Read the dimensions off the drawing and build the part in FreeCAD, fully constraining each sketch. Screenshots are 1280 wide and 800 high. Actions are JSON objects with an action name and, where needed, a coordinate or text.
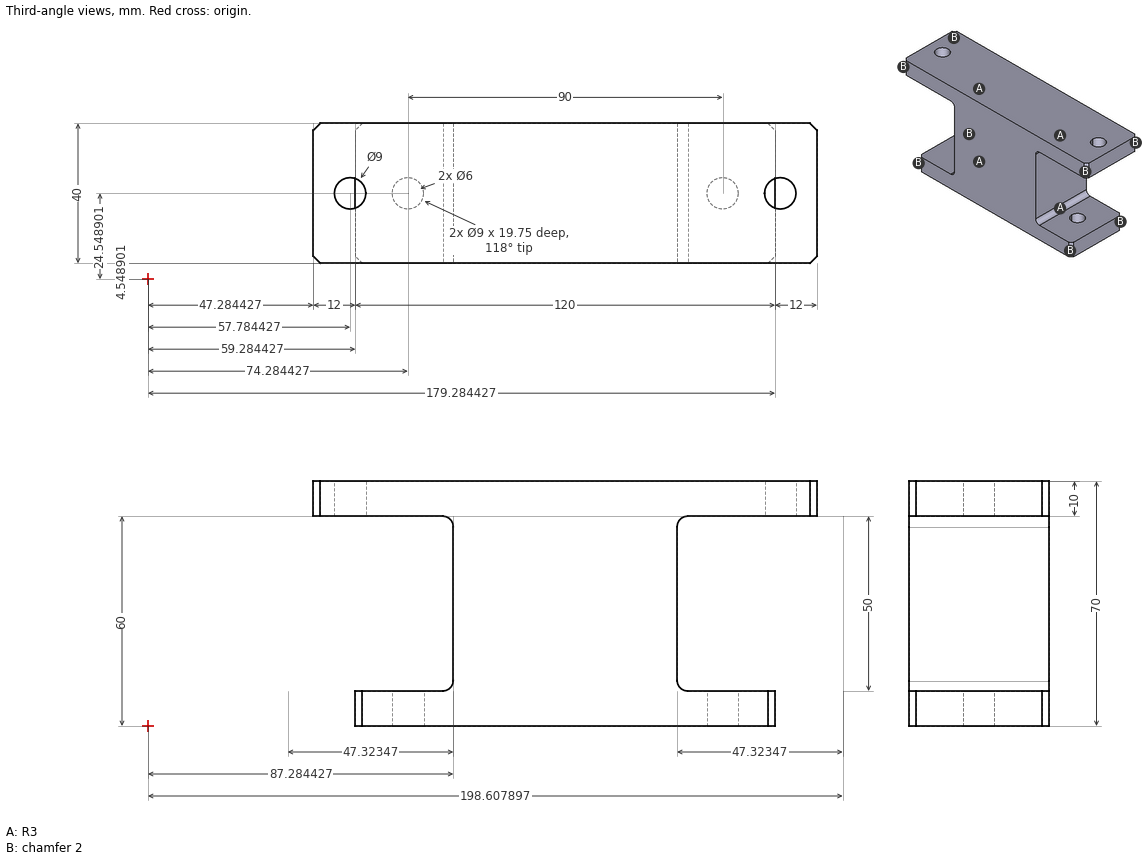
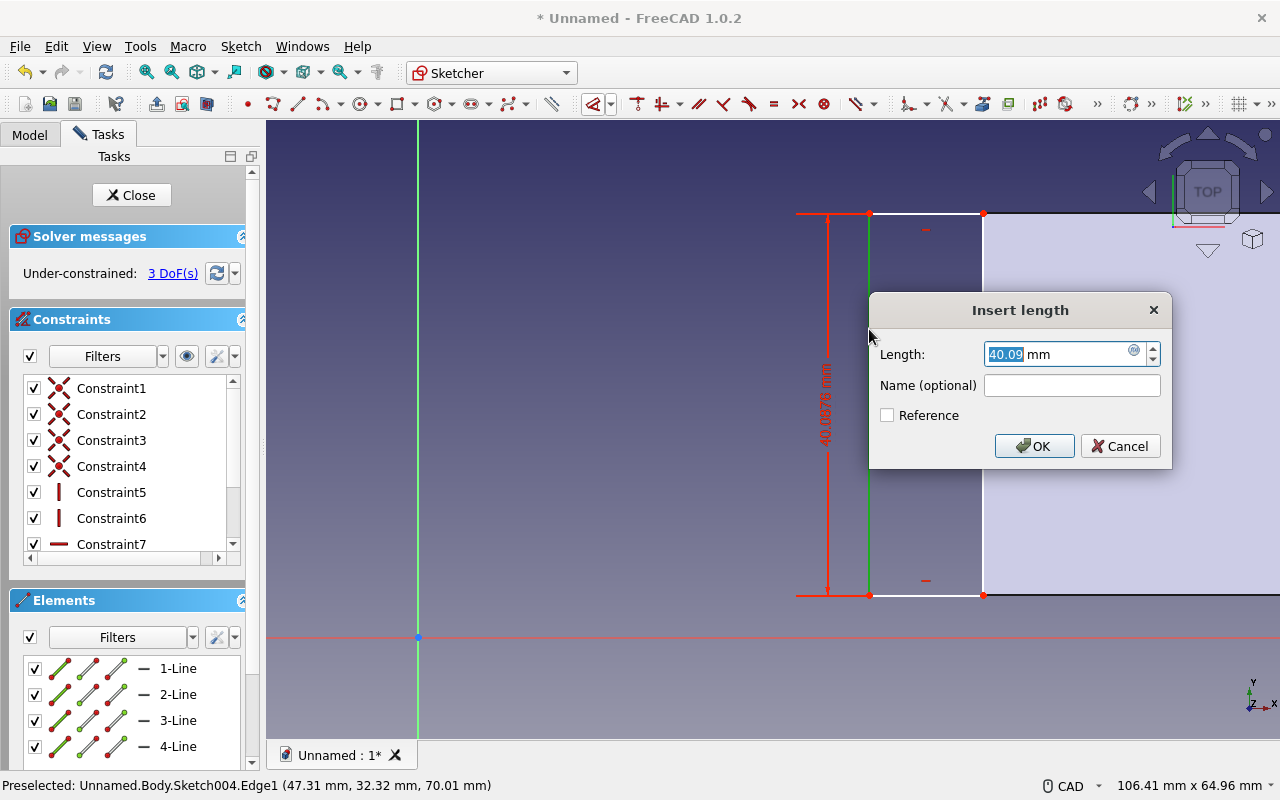
{"action": "type", "text": "40"}
{"action": "key", "text": "Return"}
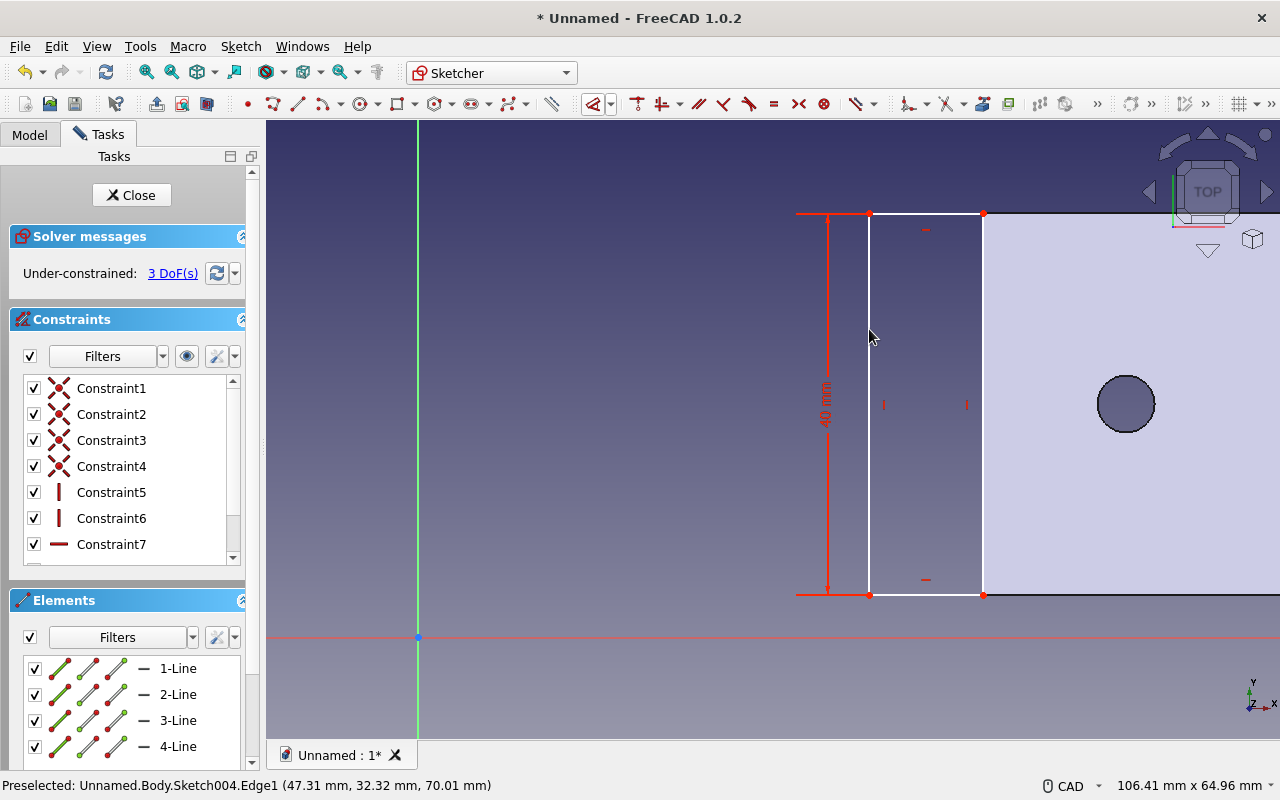
{"action": "left_click", "coordinate": [903, 595]}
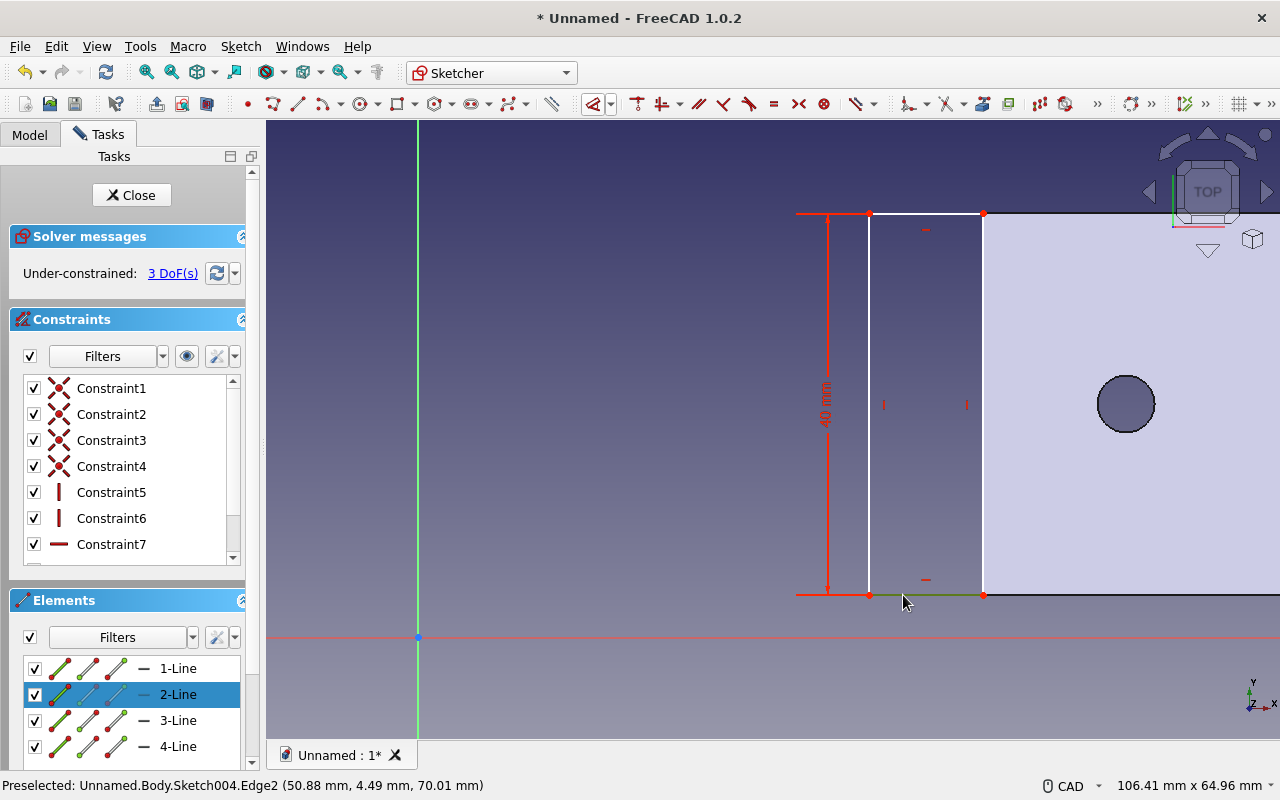
{"action": "key", "text": "l"}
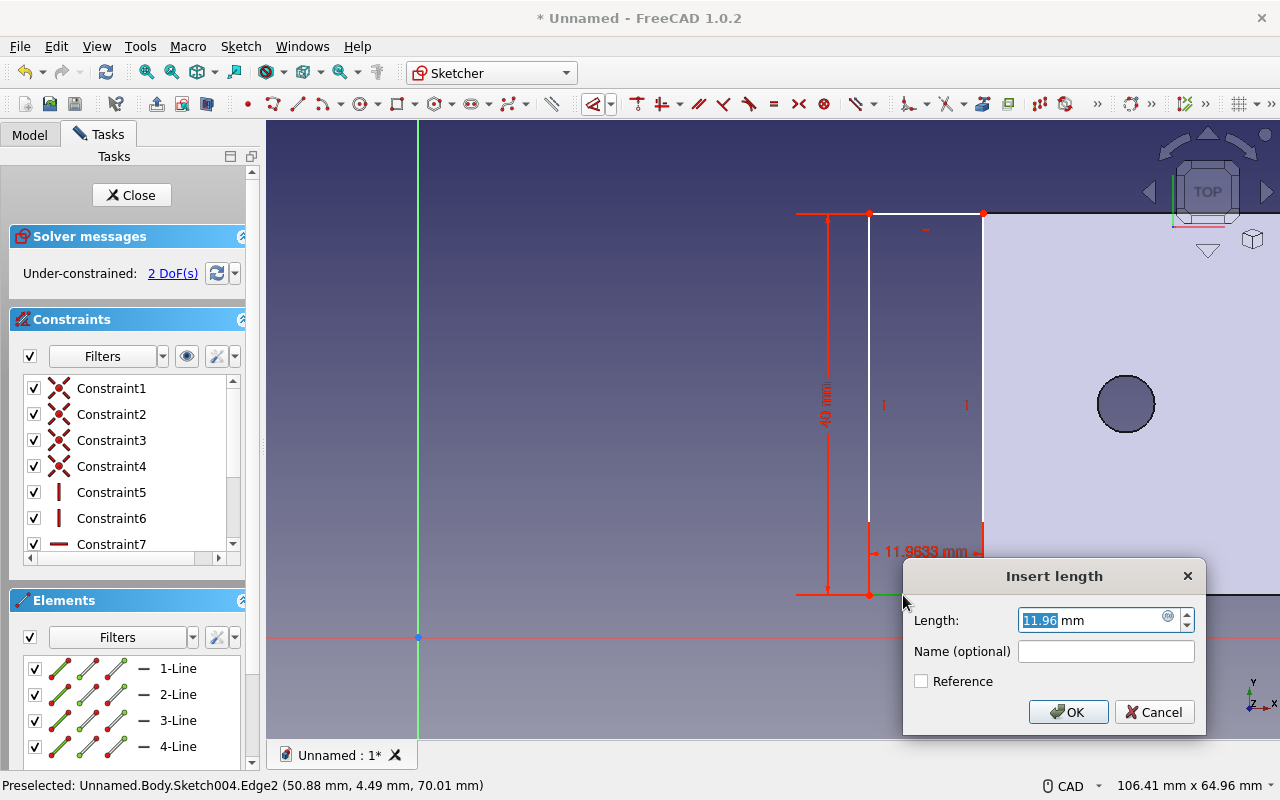
{"action": "type", "text": "12"}
{"action": "key", "text": "Return"}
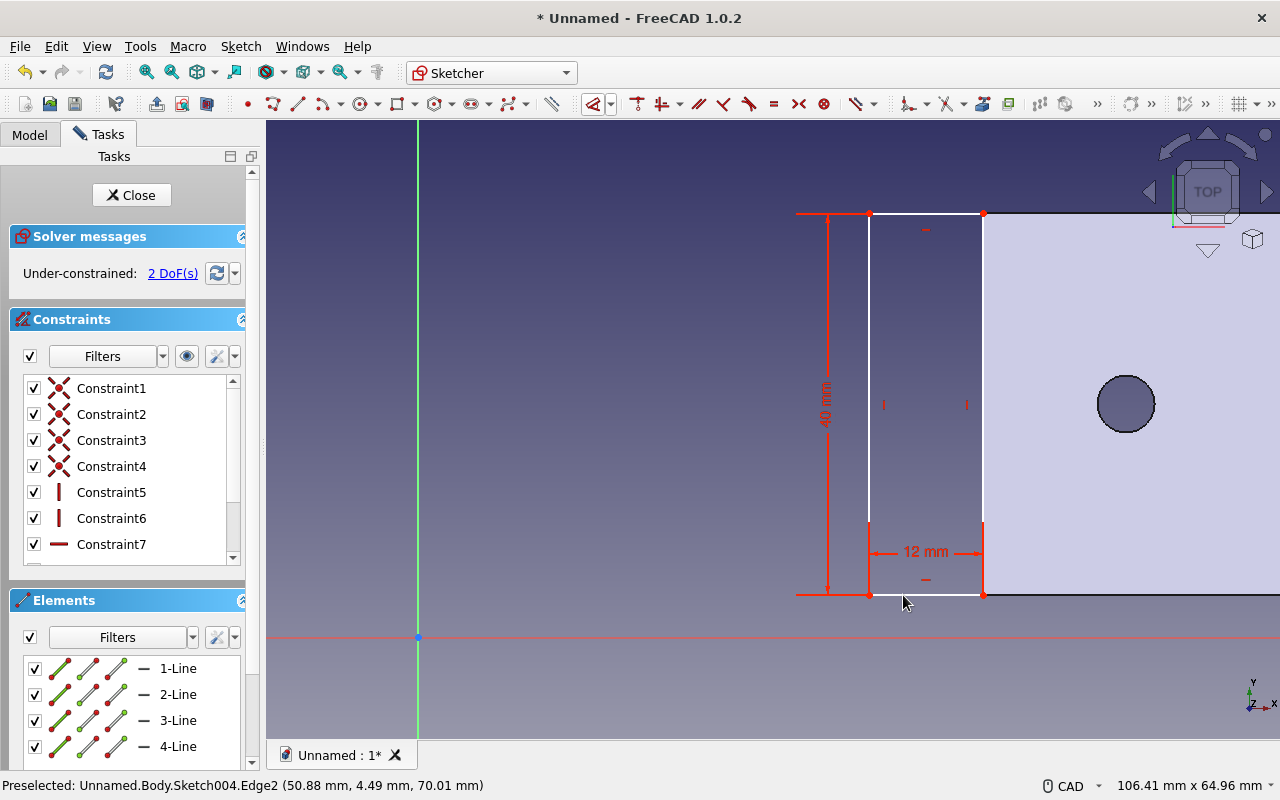
{"action": "left_click", "coordinate": [869, 595]}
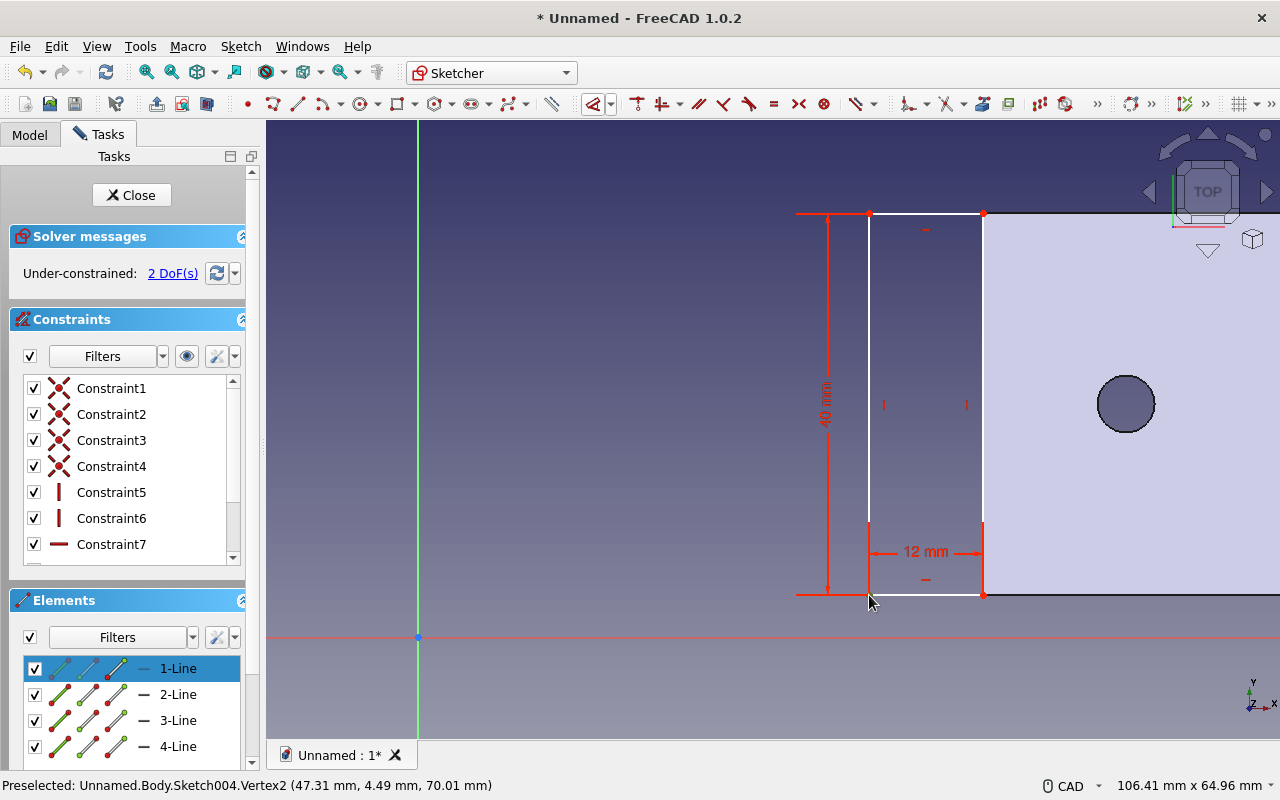
{"action": "left_click", "coordinate": [610, 104]}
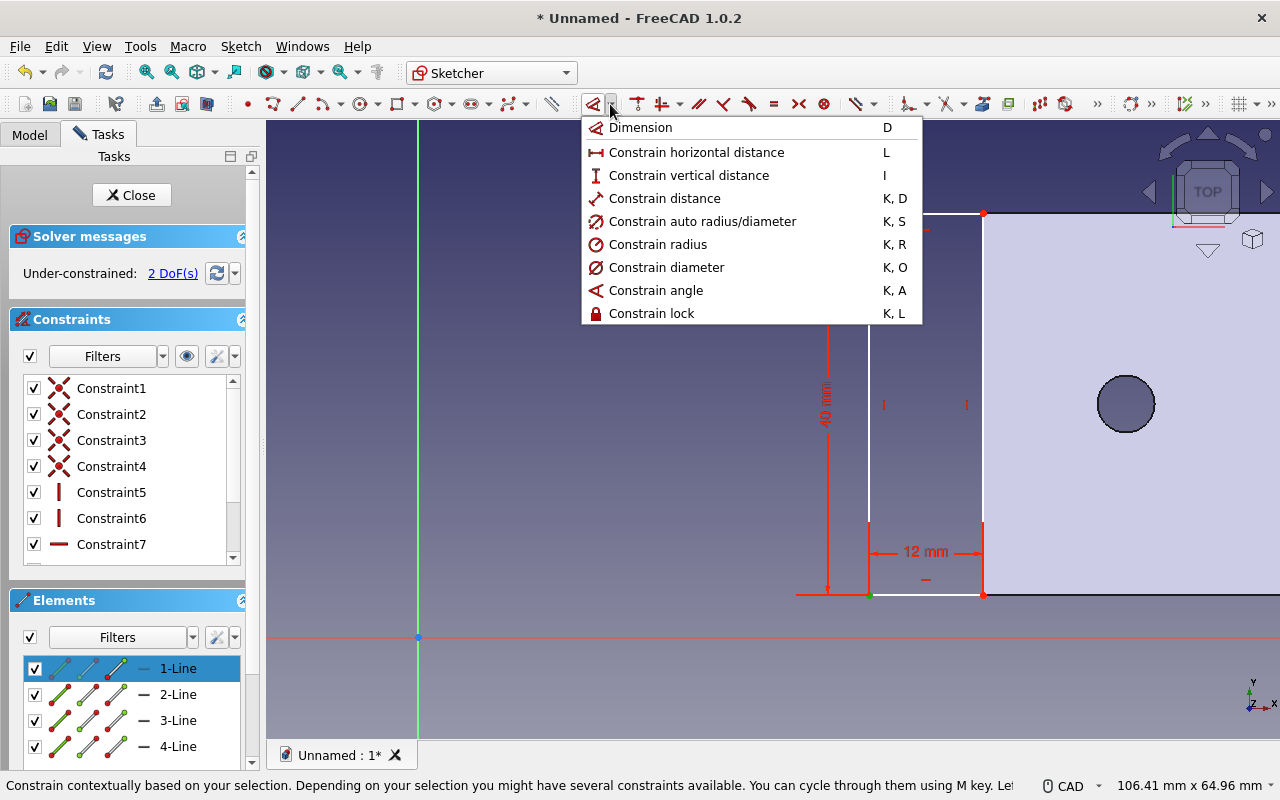
{"action": "left_click", "coordinate": [752, 176]}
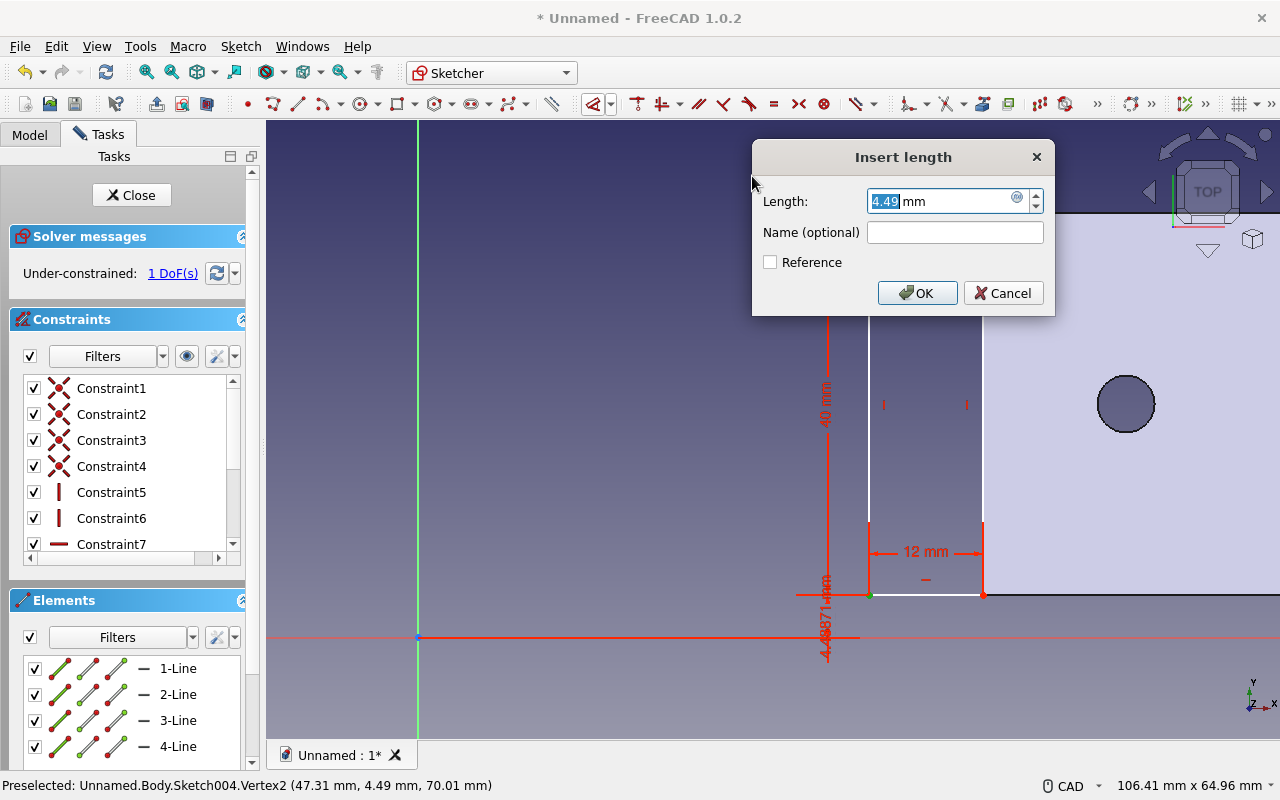
{"action": "type", "text": "4.548901"}
{"action": "key", "text": "Return"}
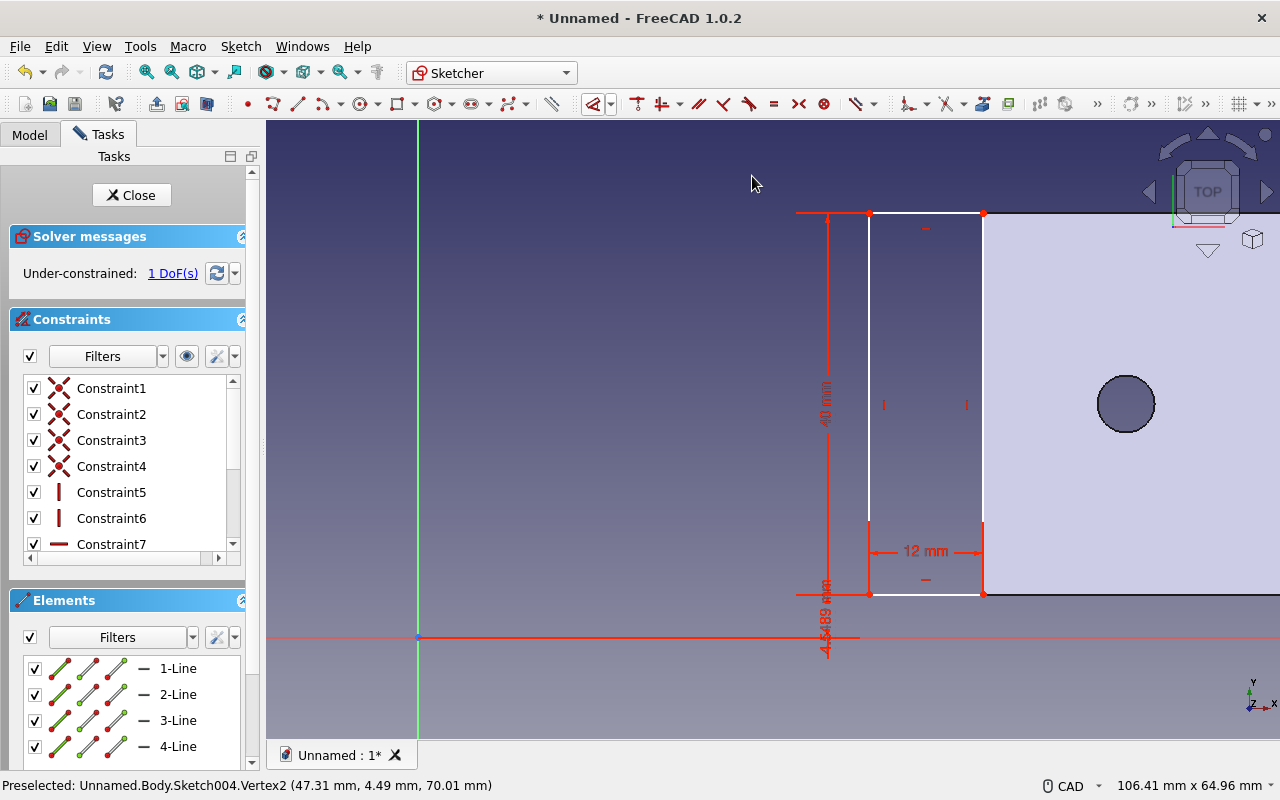
{"action": "left_click", "coordinate": [869, 213]}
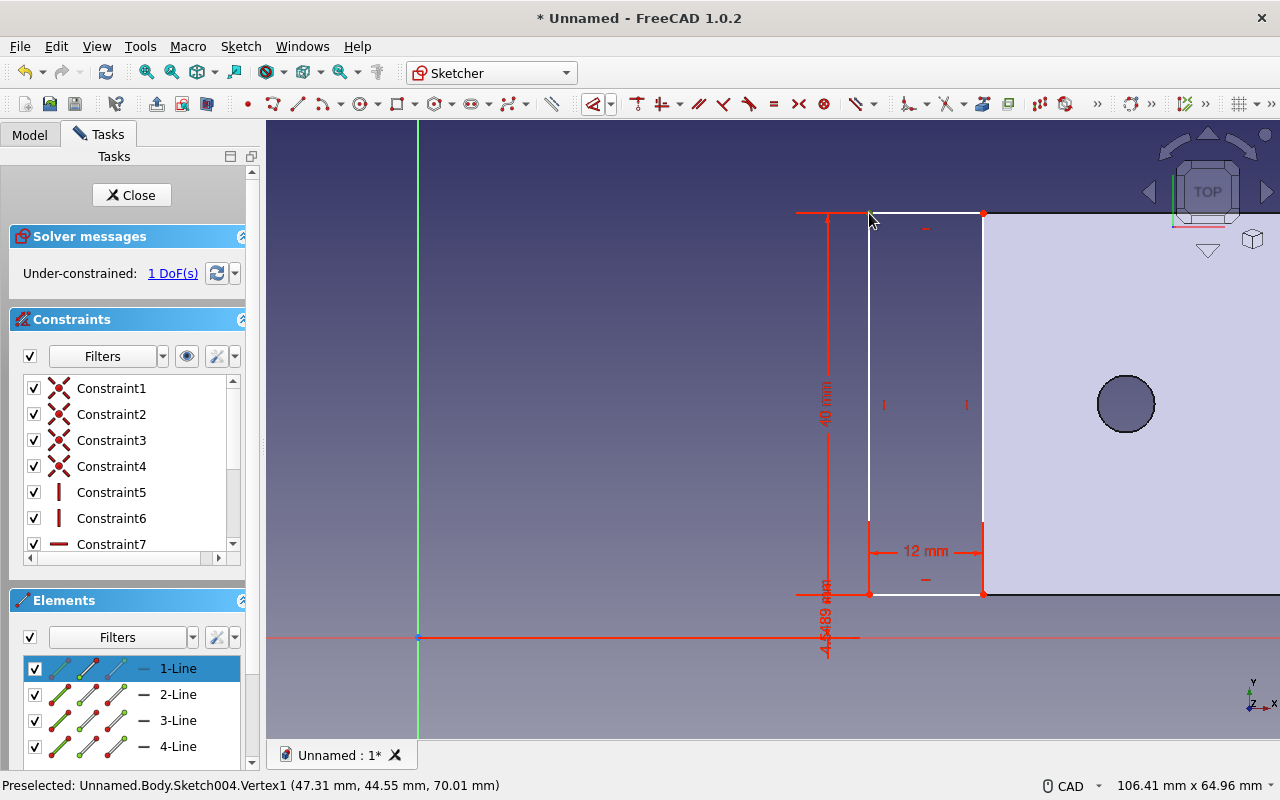
{"action": "key", "text": "l"}